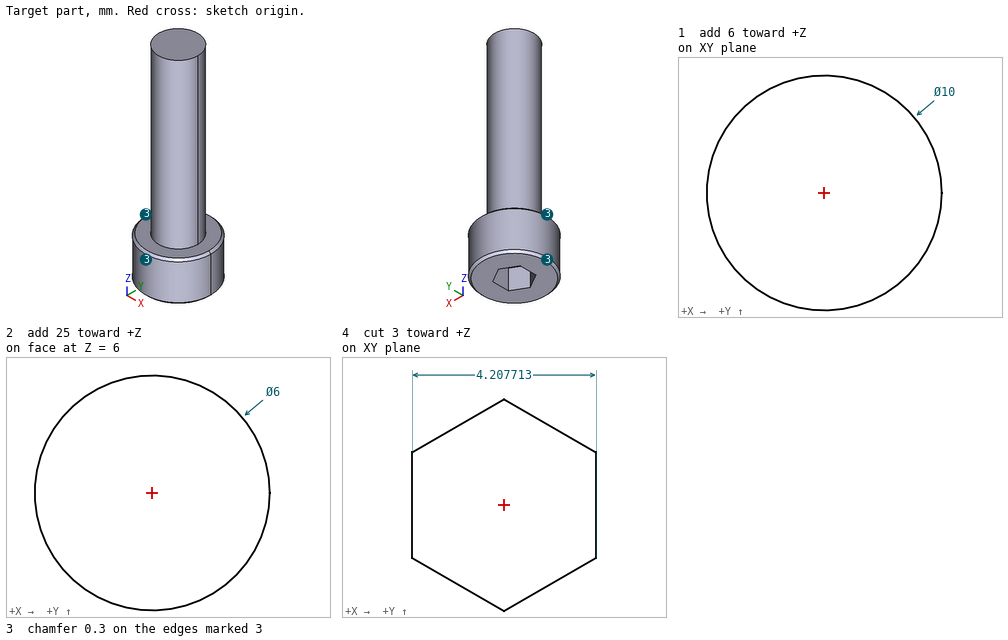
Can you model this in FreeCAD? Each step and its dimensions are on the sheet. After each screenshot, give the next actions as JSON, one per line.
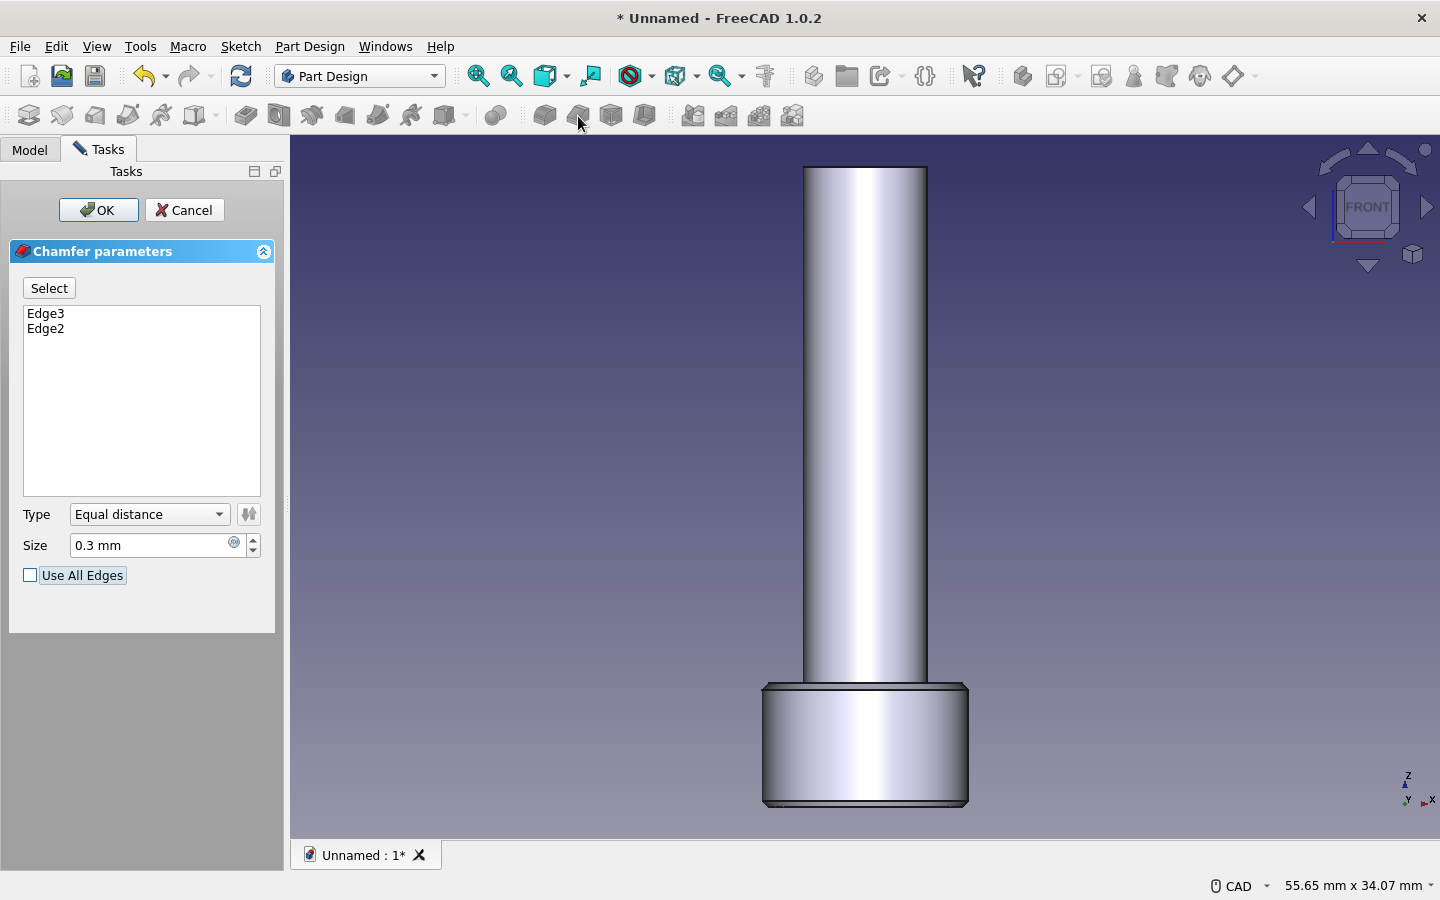
{"action": "left_click", "coordinate": [99, 210]}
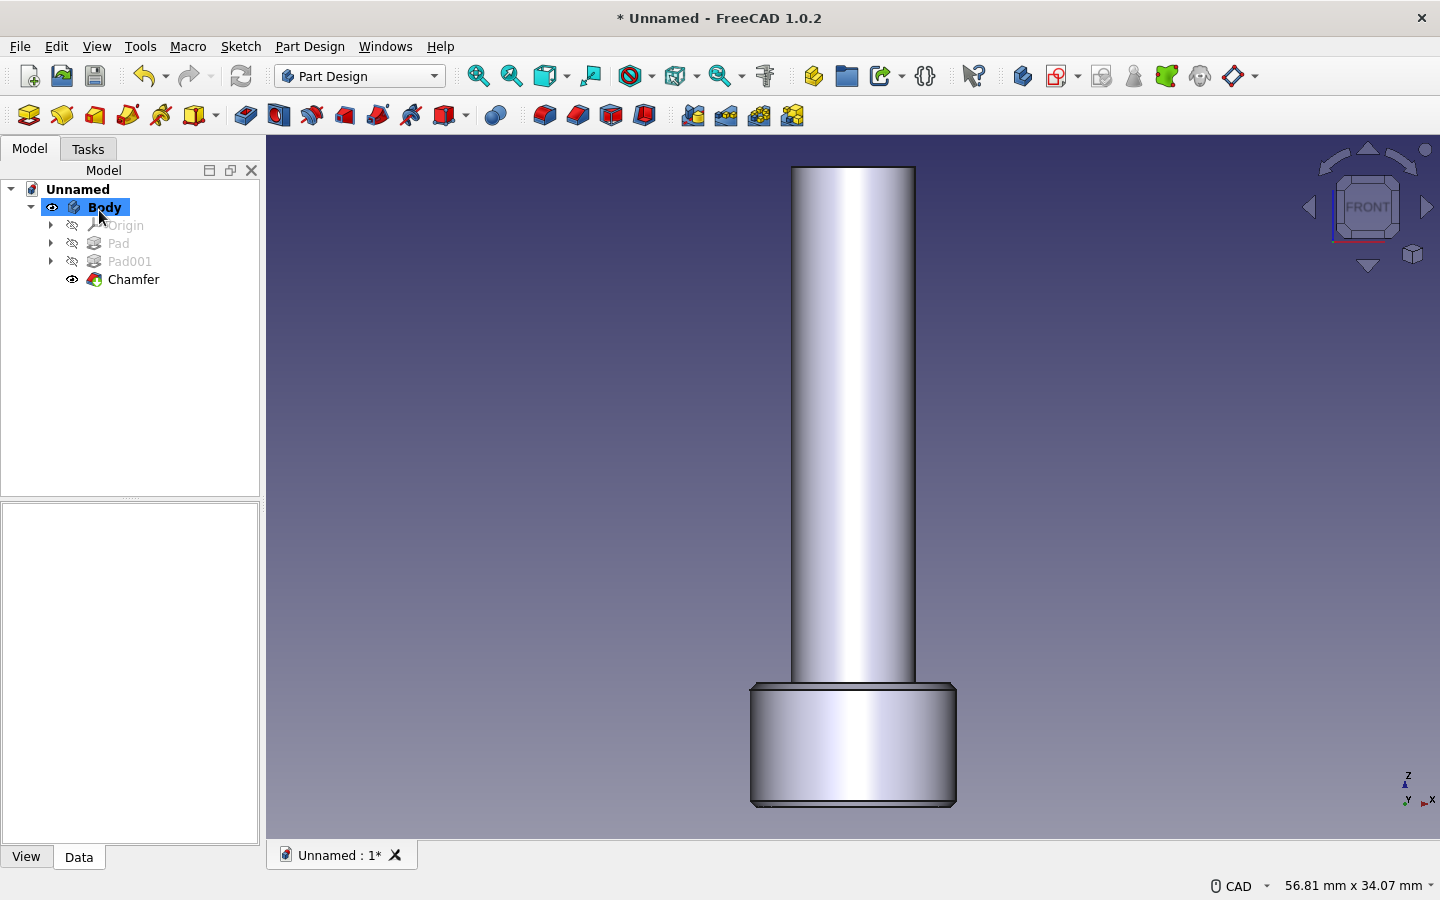
{"action": "left_click", "coordinate": [1056, 76]}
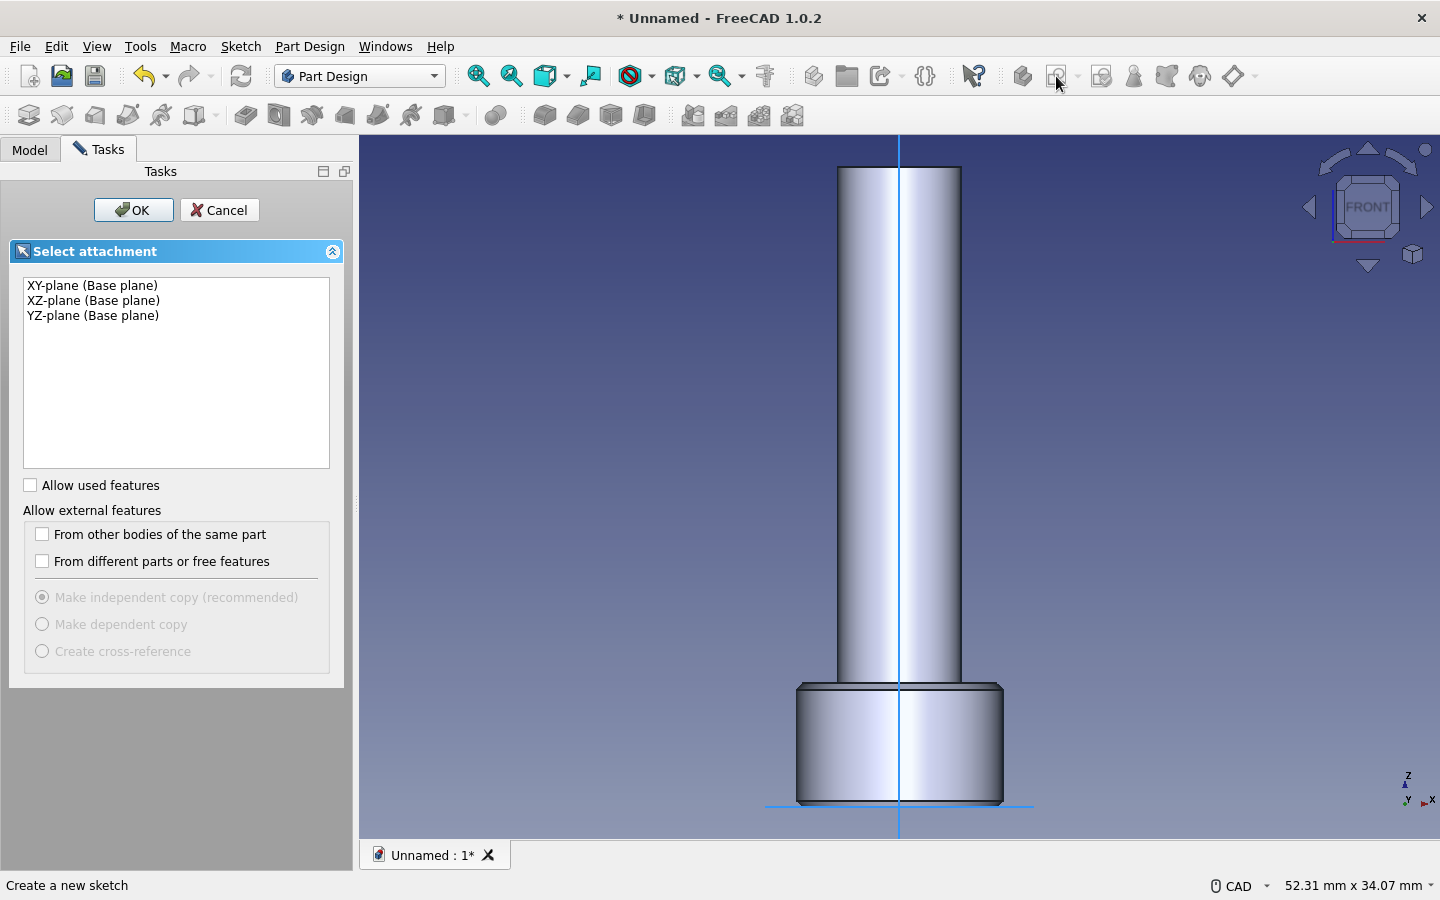
{"action": "left_click", "coordinate": [84, 286]}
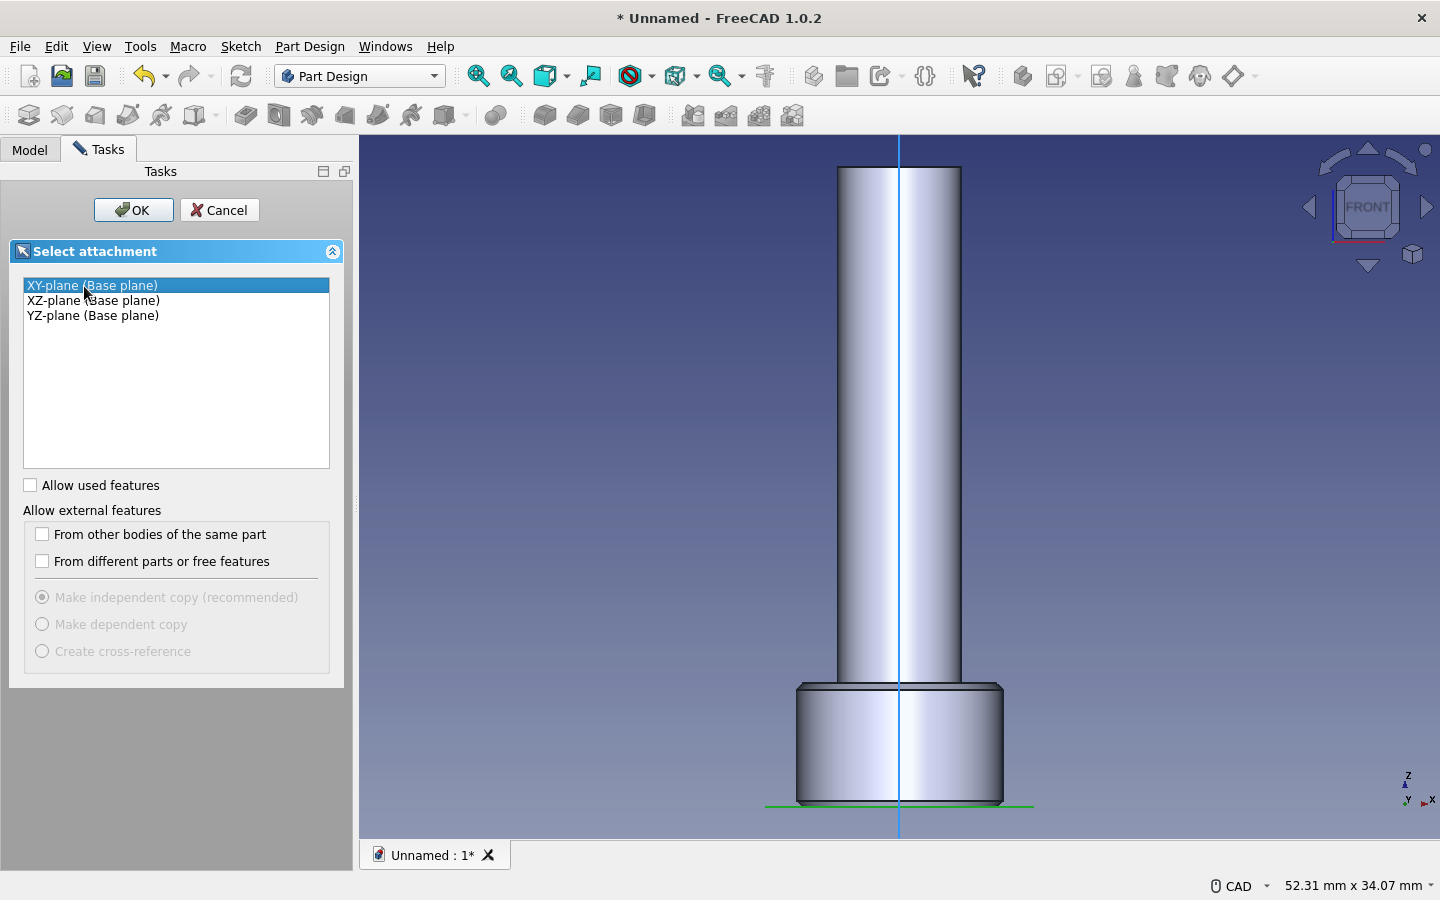
{"action": "left_click", "coordinate": [134, 210]}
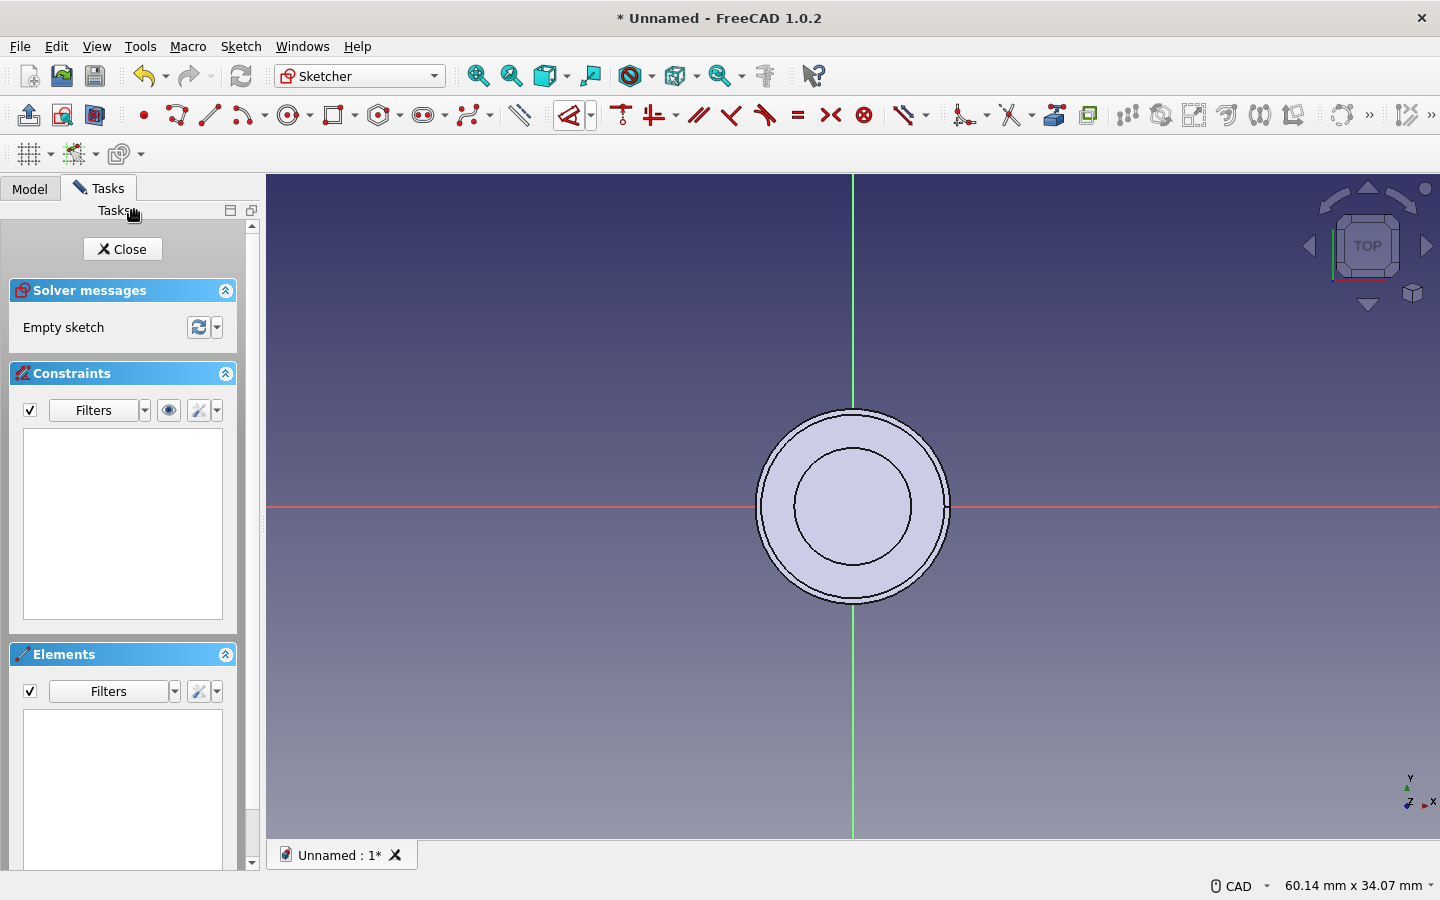
{"action": "left_click", "coordinate": [95, 116]}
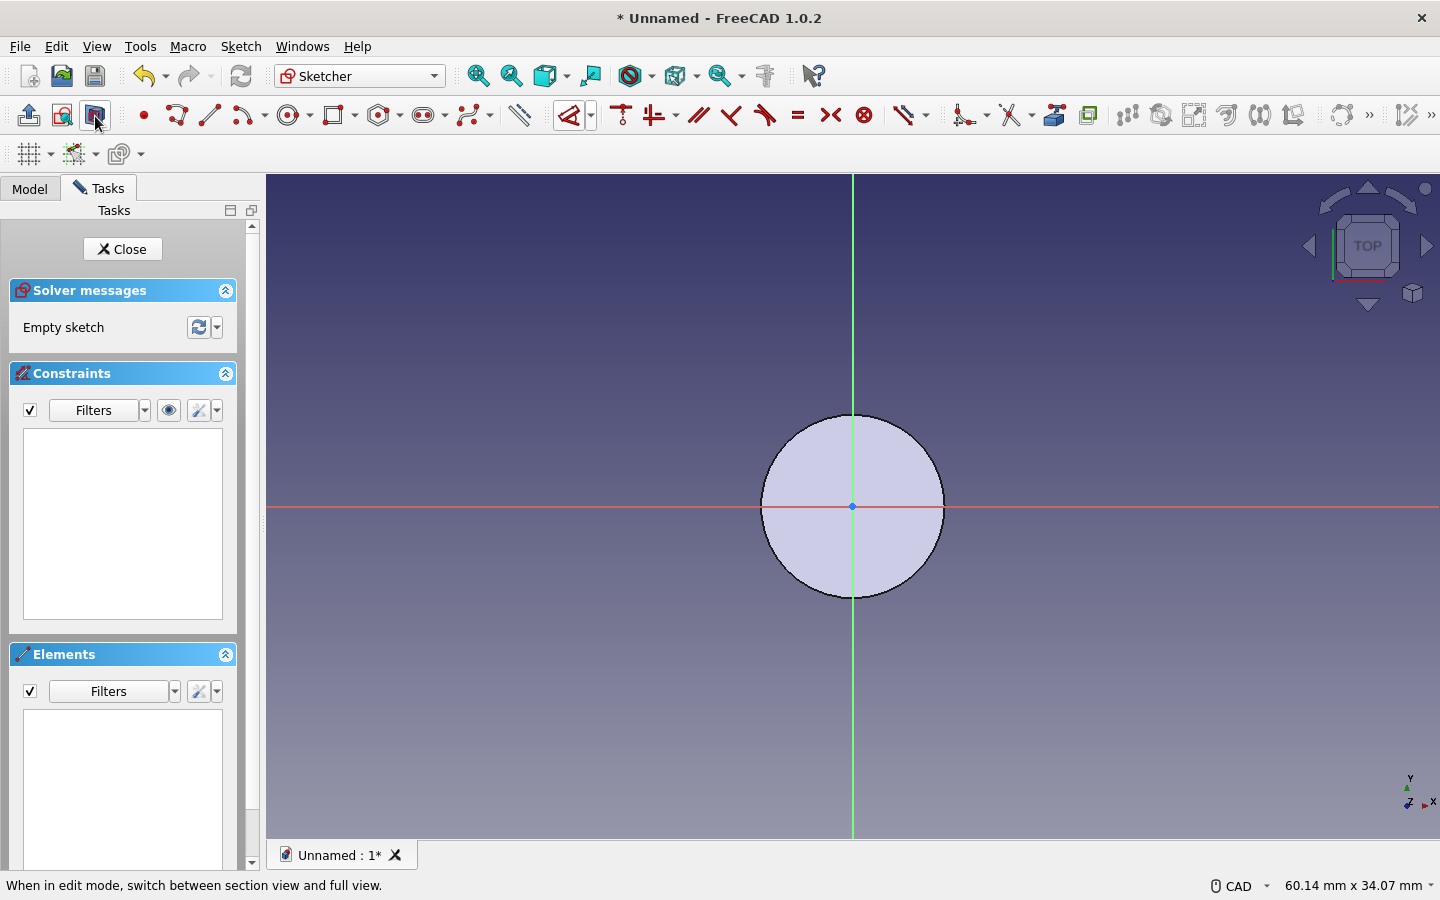
{"action": "scroll", "coordinate": [870, 506], "scroll_direction": "up", "scroll_amount": 8}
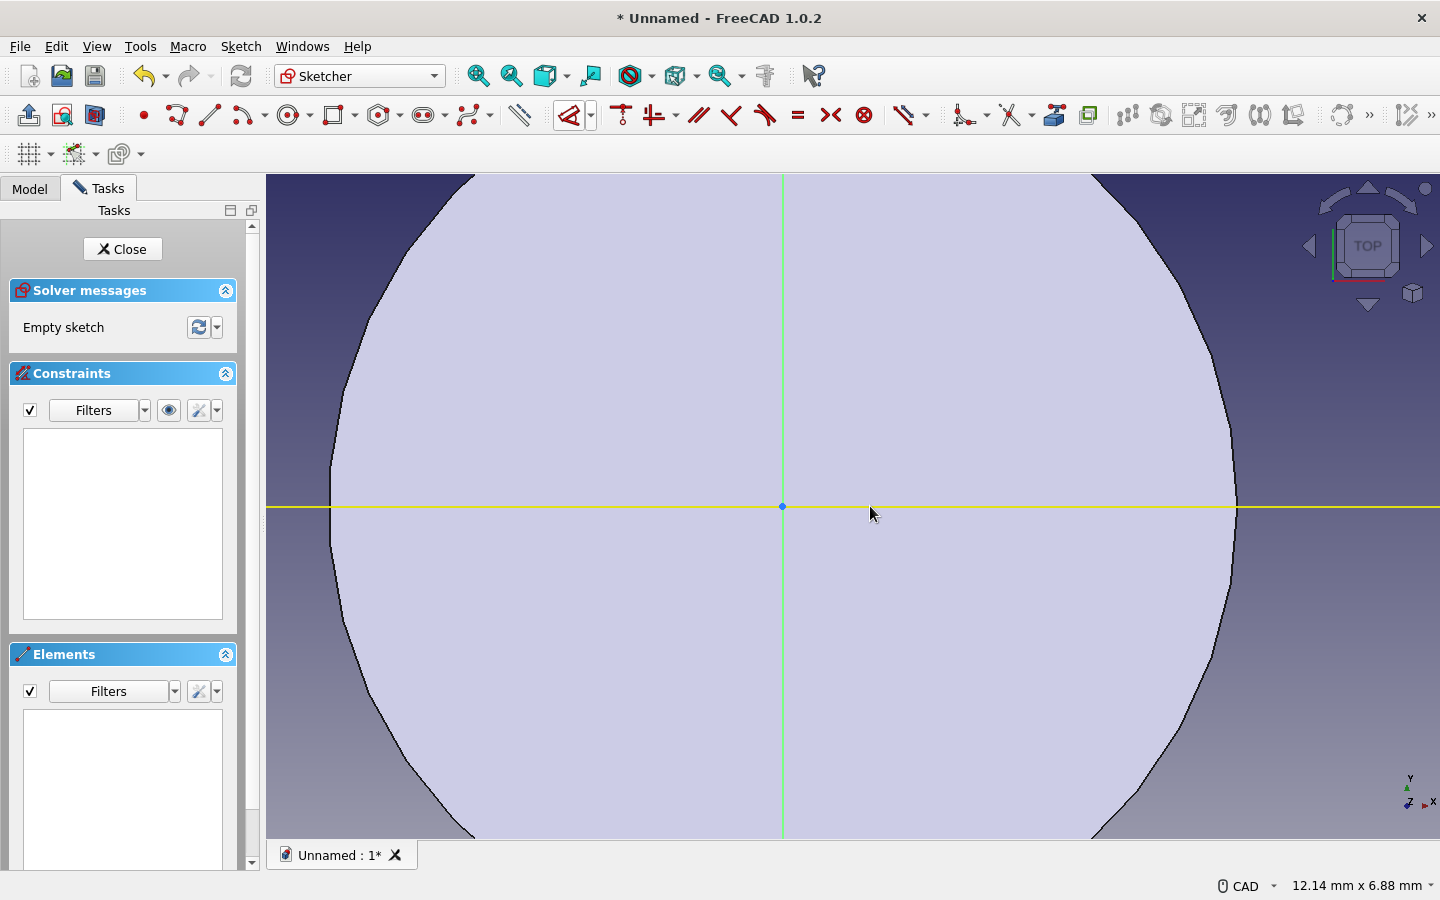
{"action": "left_click", "coordinate": [378, 116]}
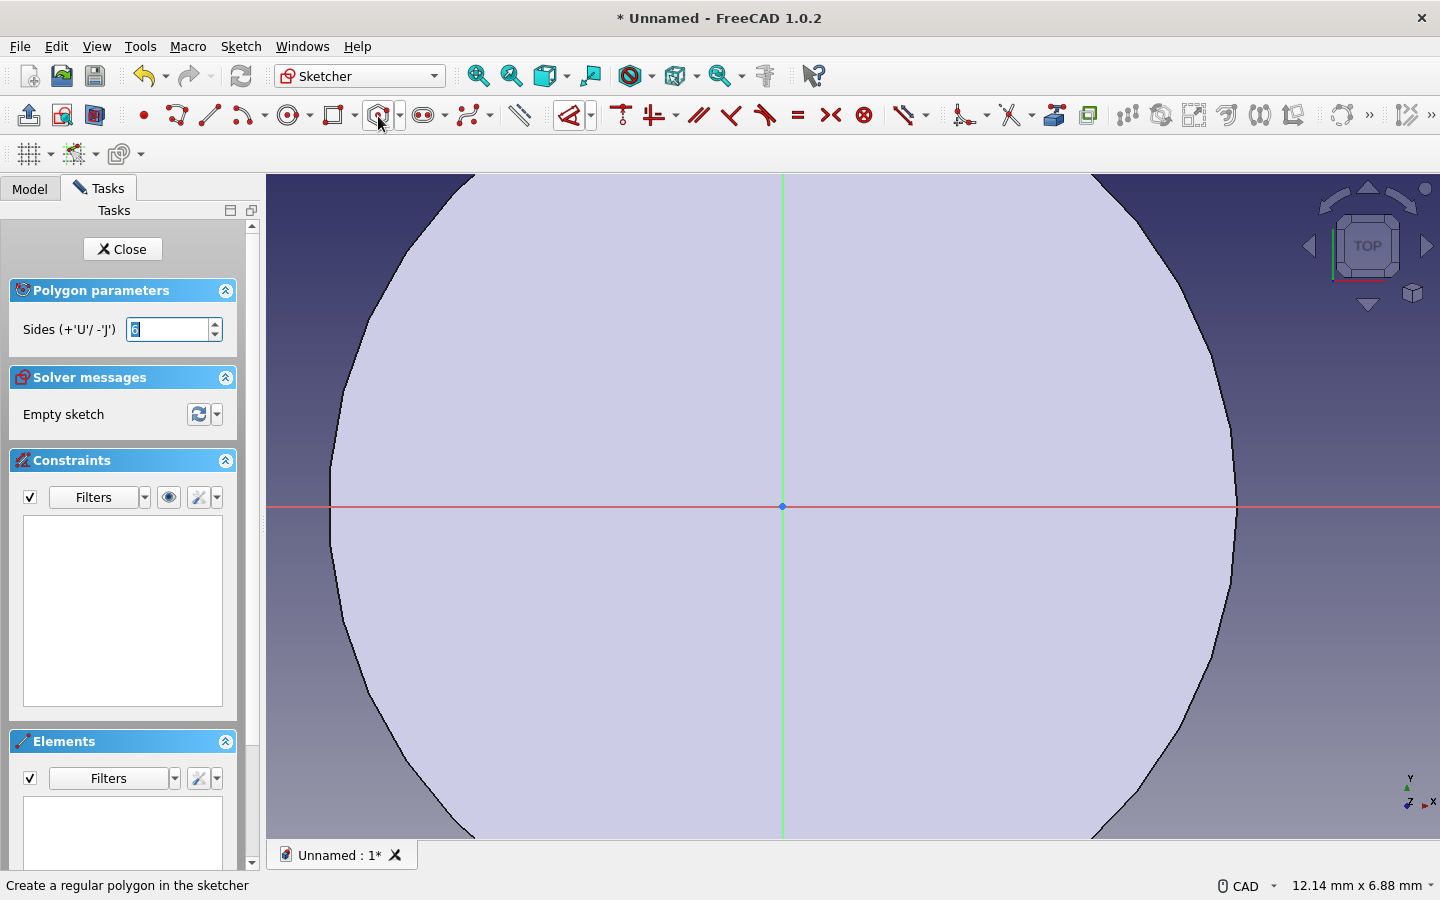
{"action": "left_click", "coordinate": [783, 506]}